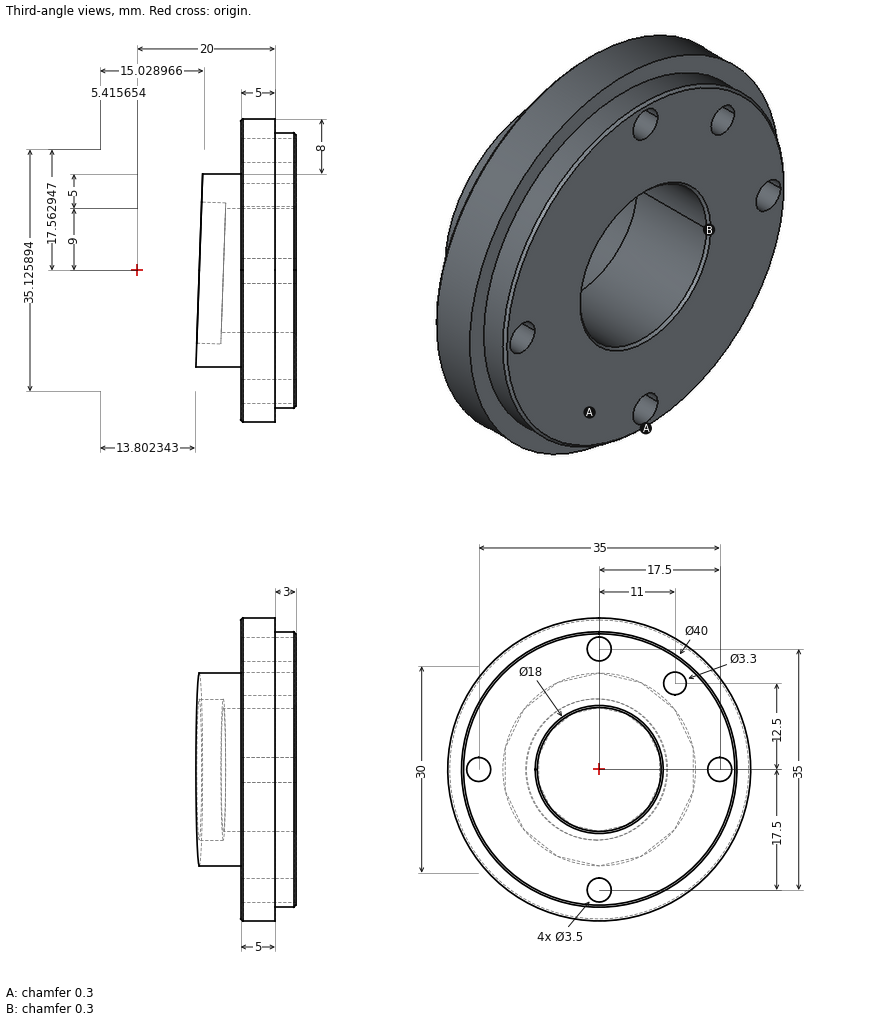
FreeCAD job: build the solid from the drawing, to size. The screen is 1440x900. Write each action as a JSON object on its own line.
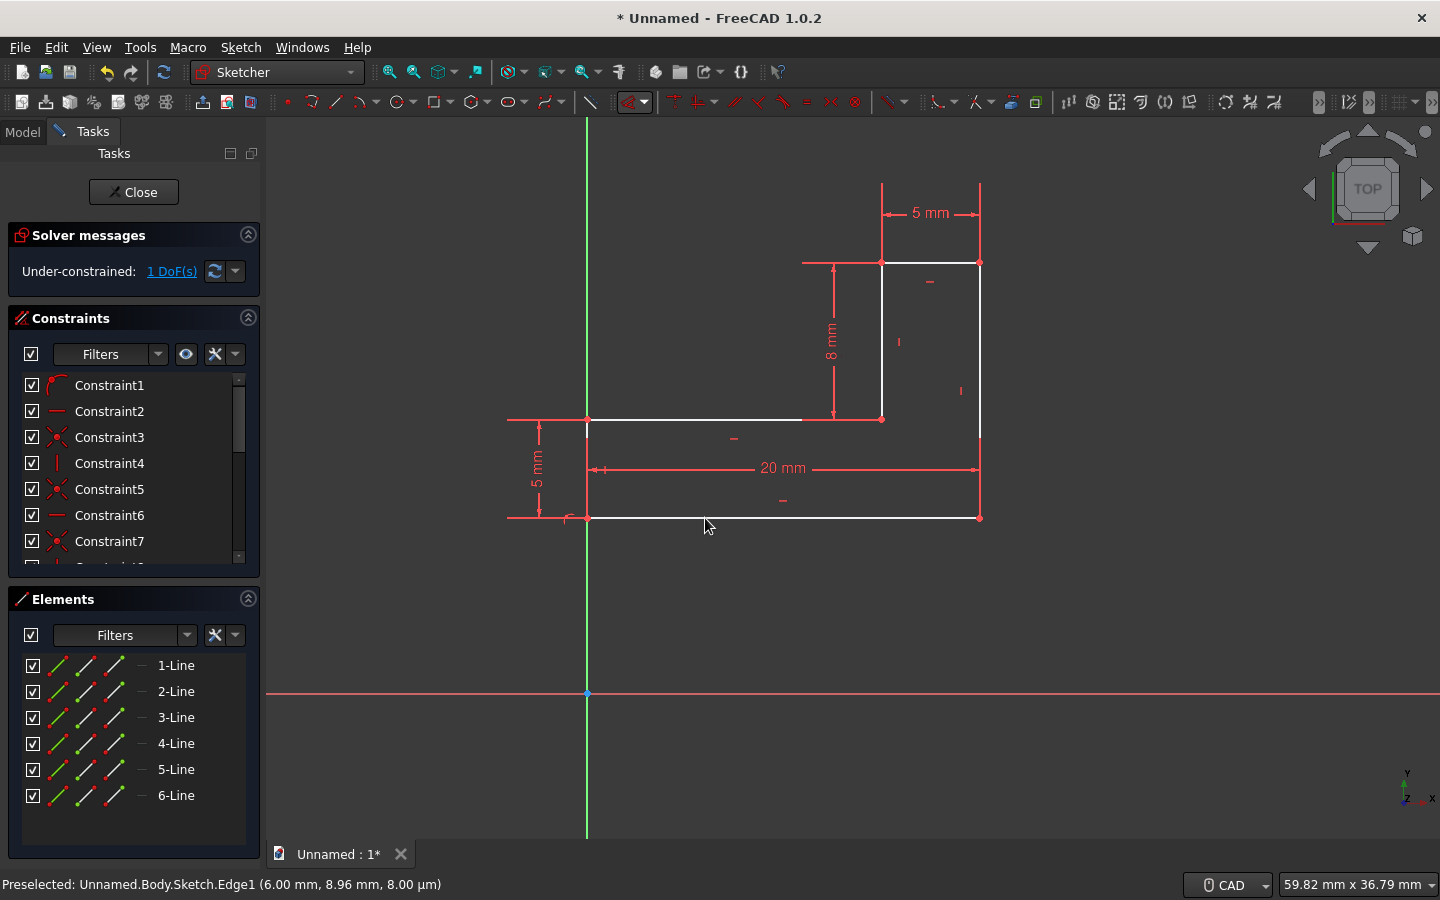
{"action": "left_click", "coordinate": [587, 518]}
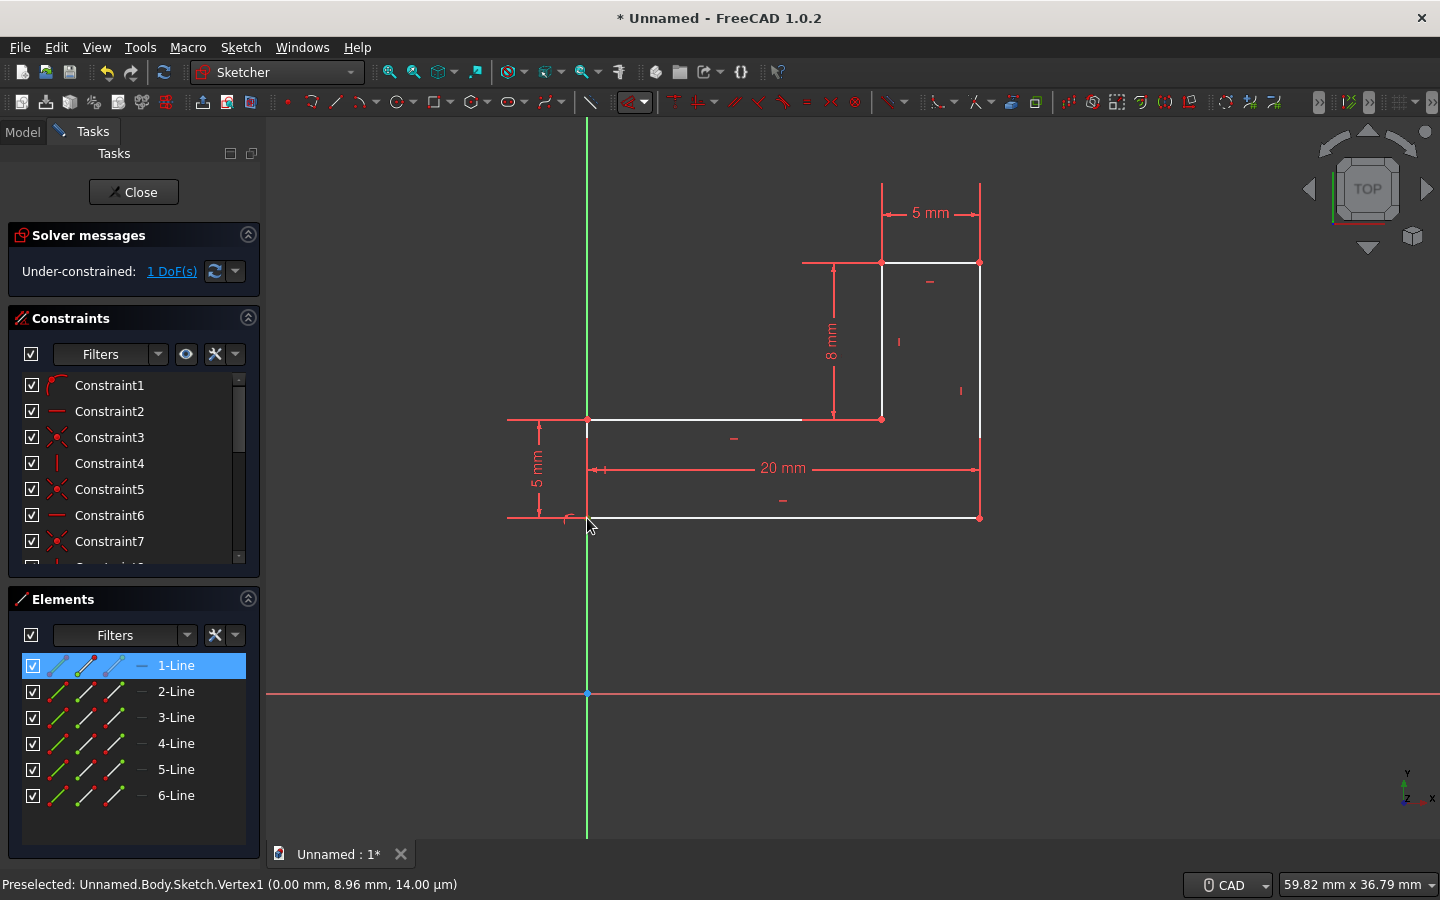
{"action": "left_click", "coordinate": [646, 102]}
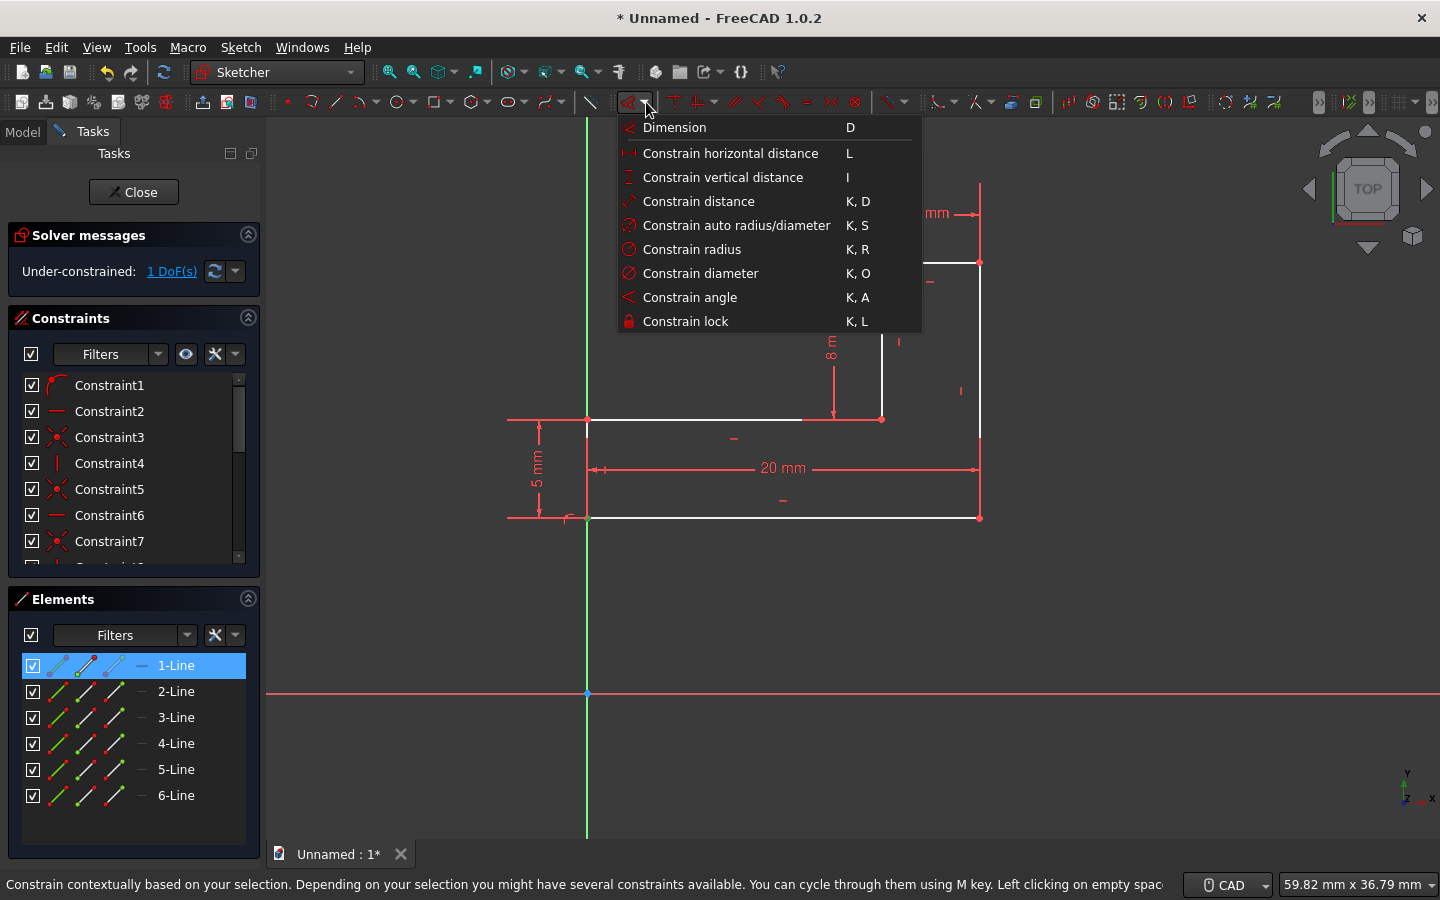
{"action": "left_click", "coordinate": [770, 177]}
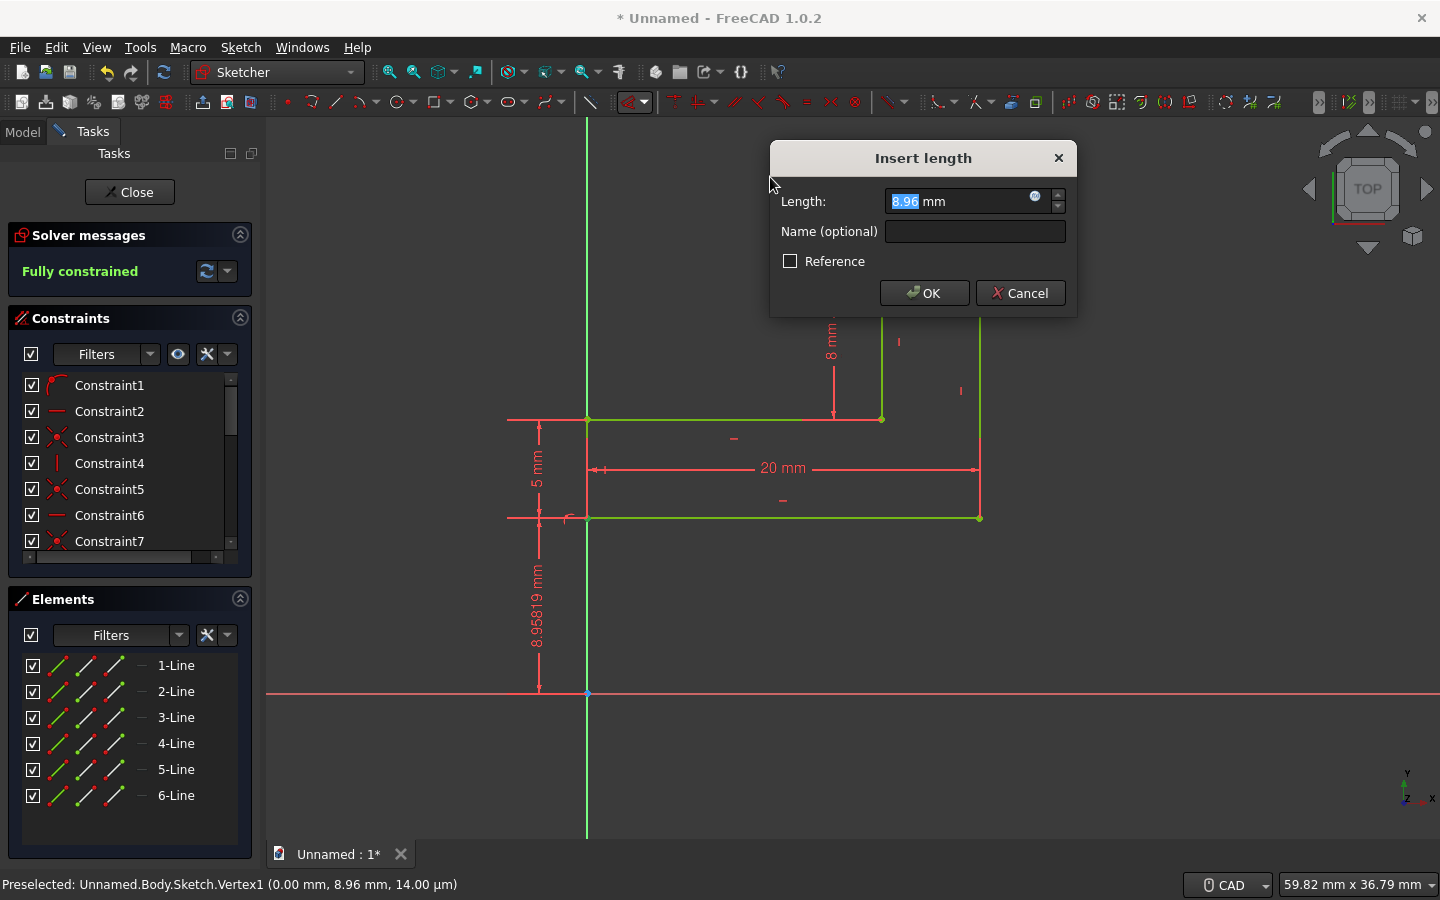
{"action": "type", "text": "9"}
{"action": "key", "text": "Return"}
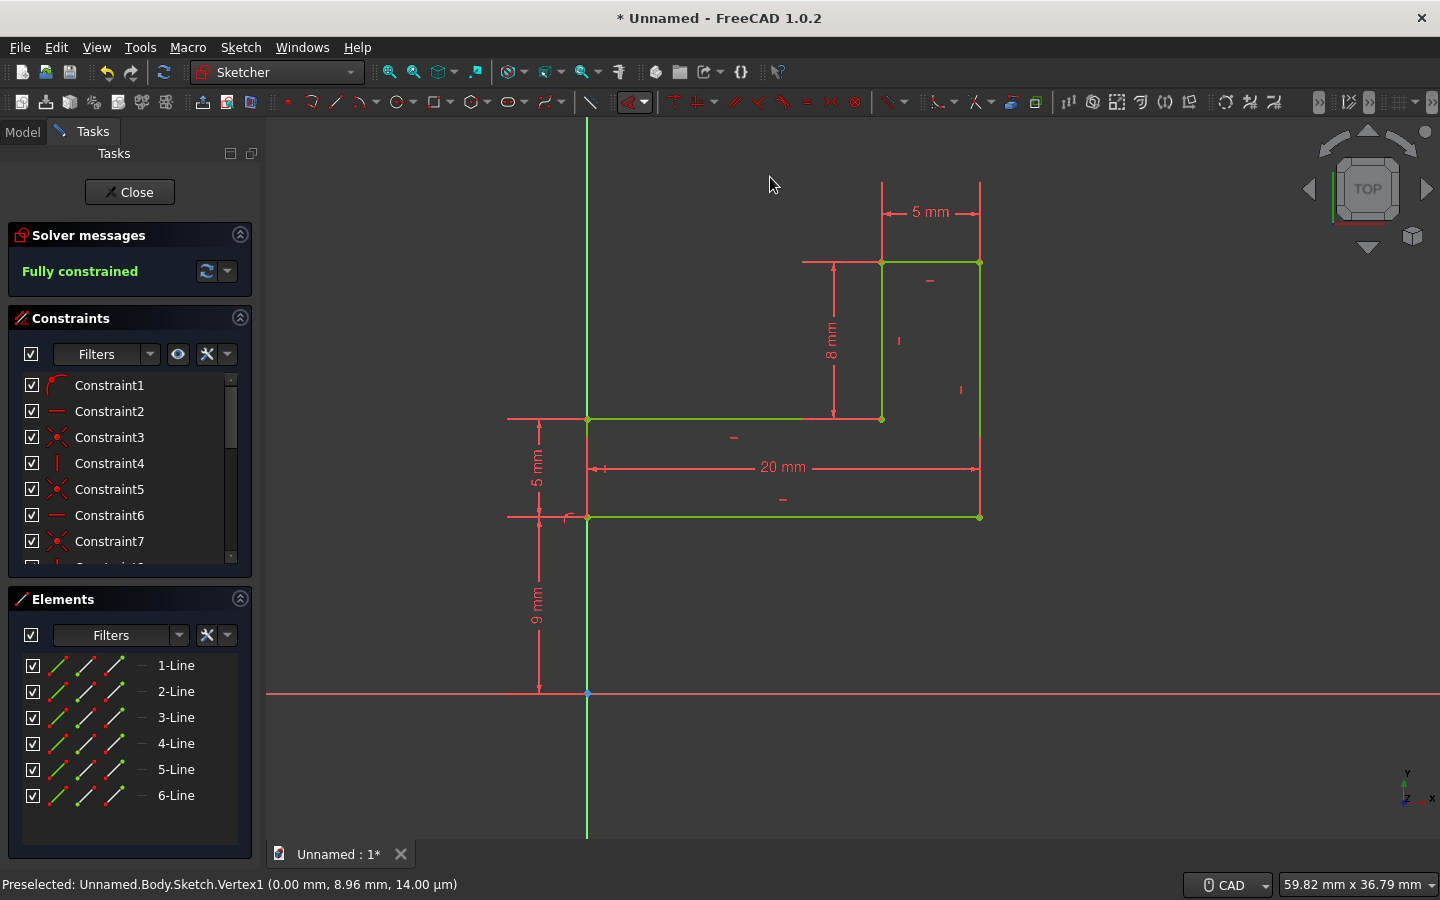
{"action": "left_click", "coordinate": [130, 192]}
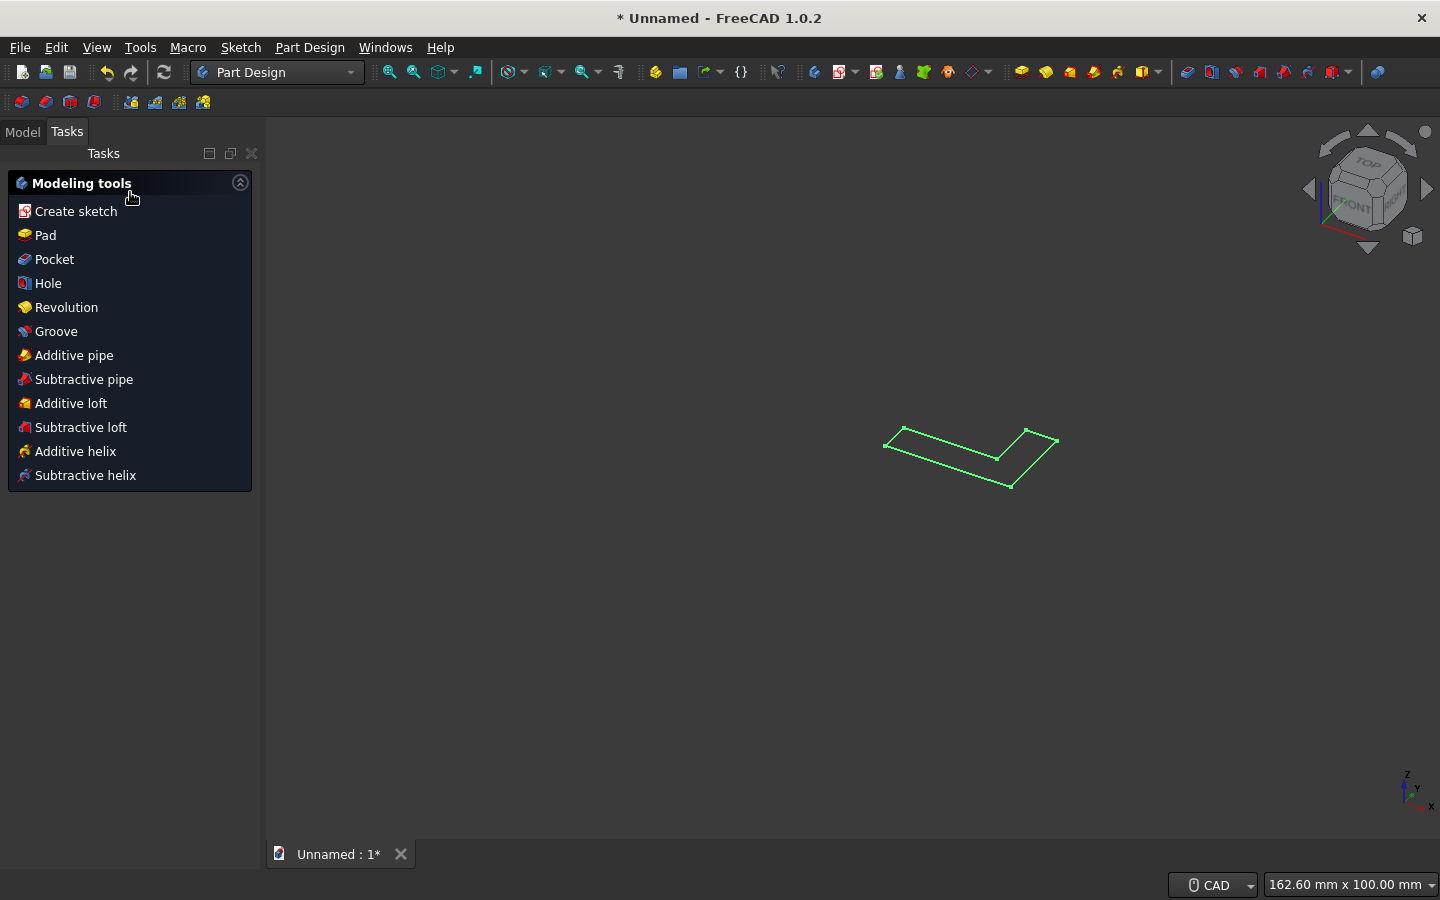
{"action": "left_click", "coordinate": [1046, 72]}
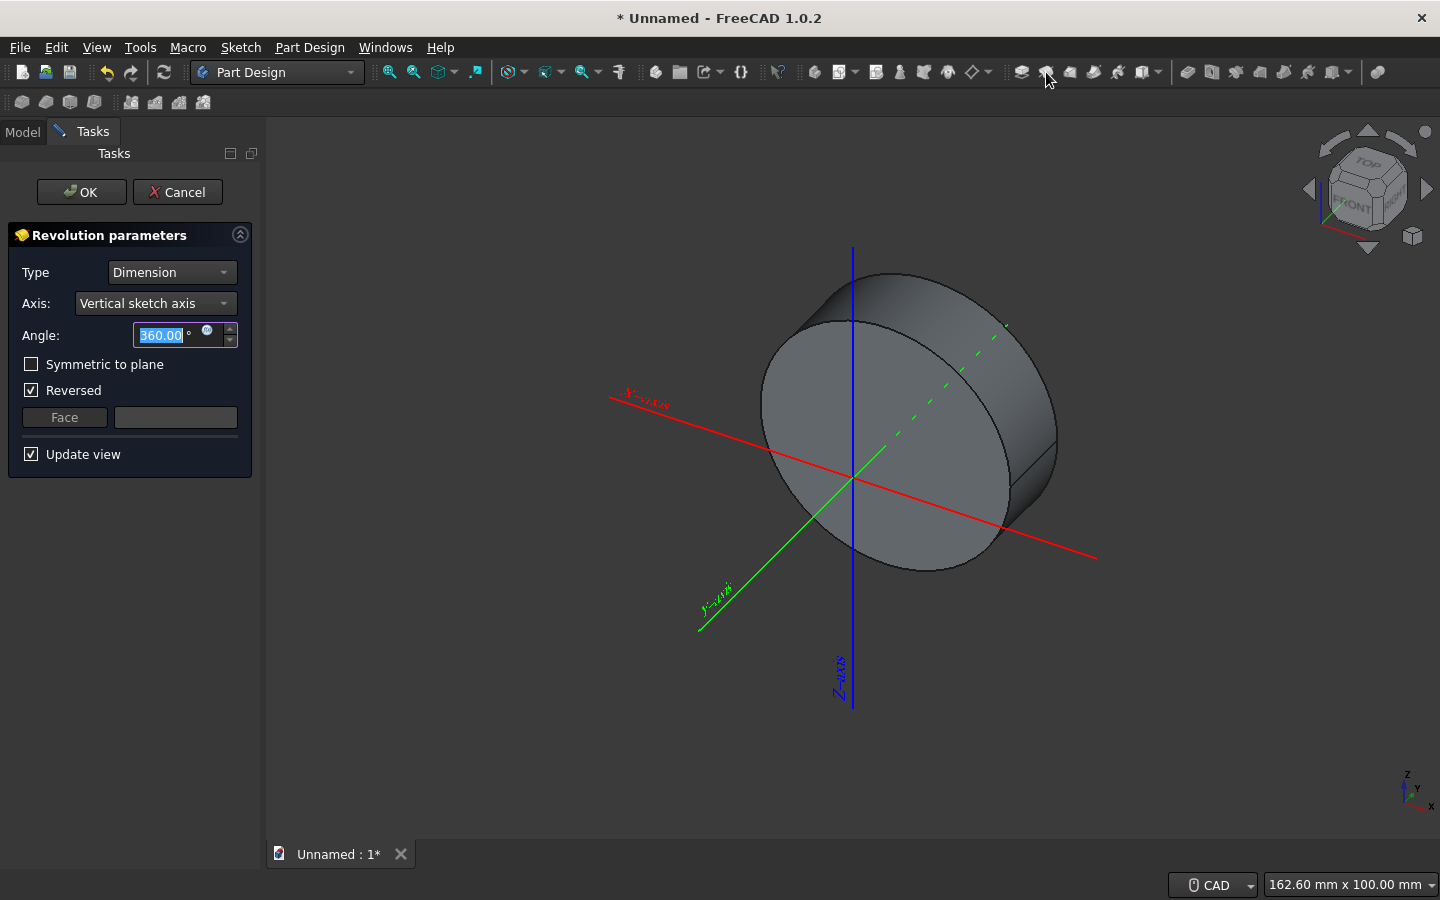
{"action": "left_click", "coordinate": [156, 304]}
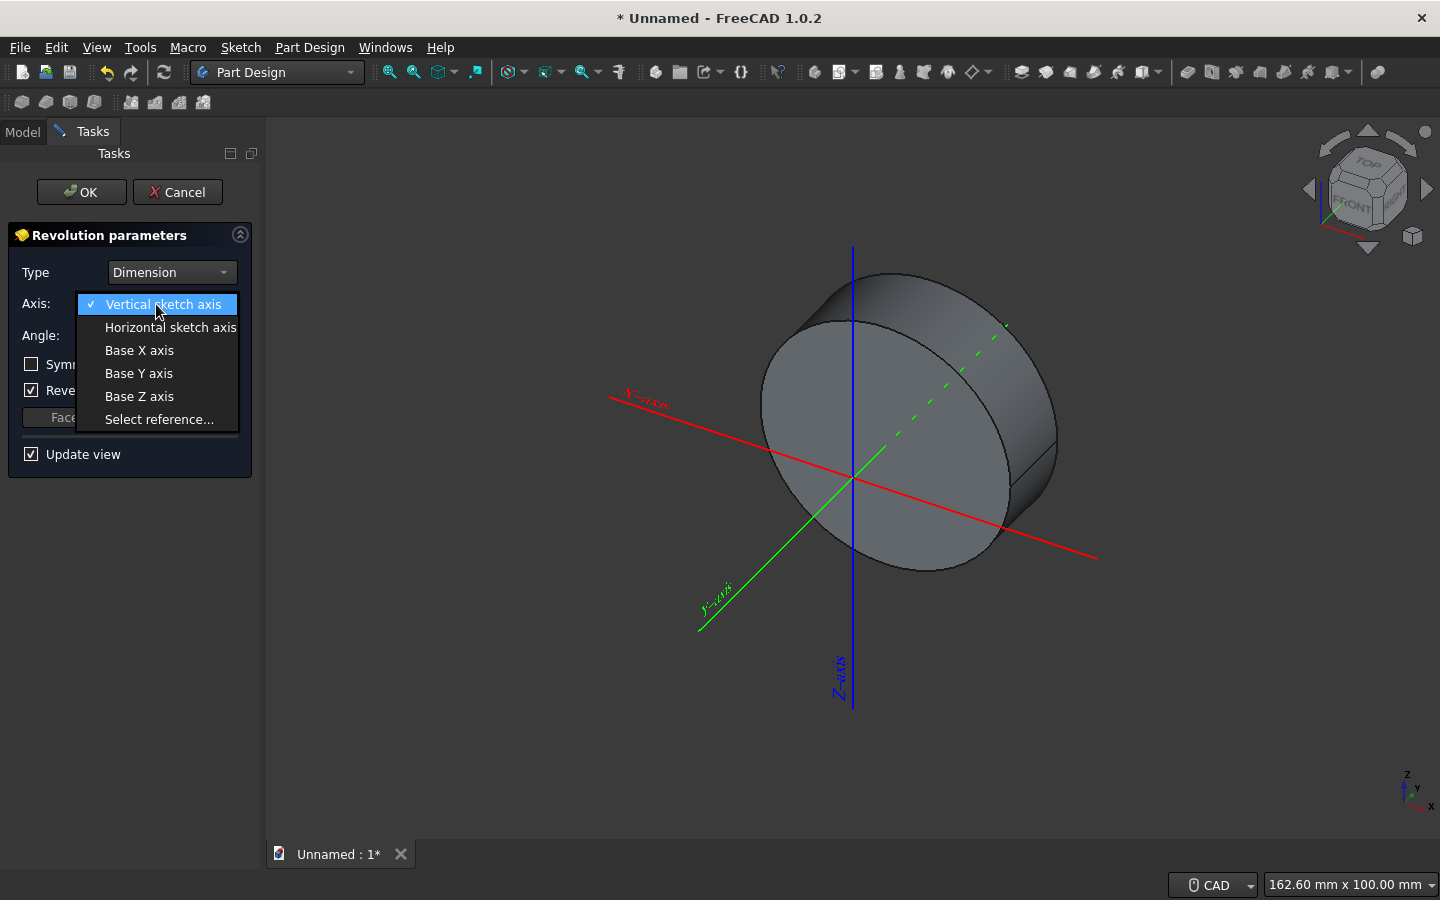
{"action": "left_click", "coordinate": [156, 328]}